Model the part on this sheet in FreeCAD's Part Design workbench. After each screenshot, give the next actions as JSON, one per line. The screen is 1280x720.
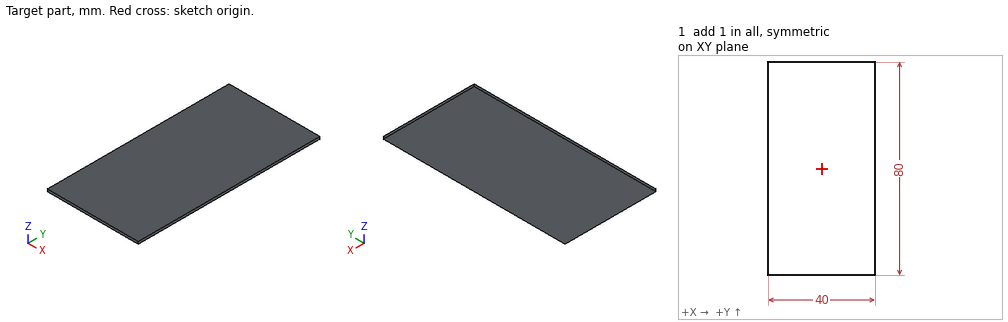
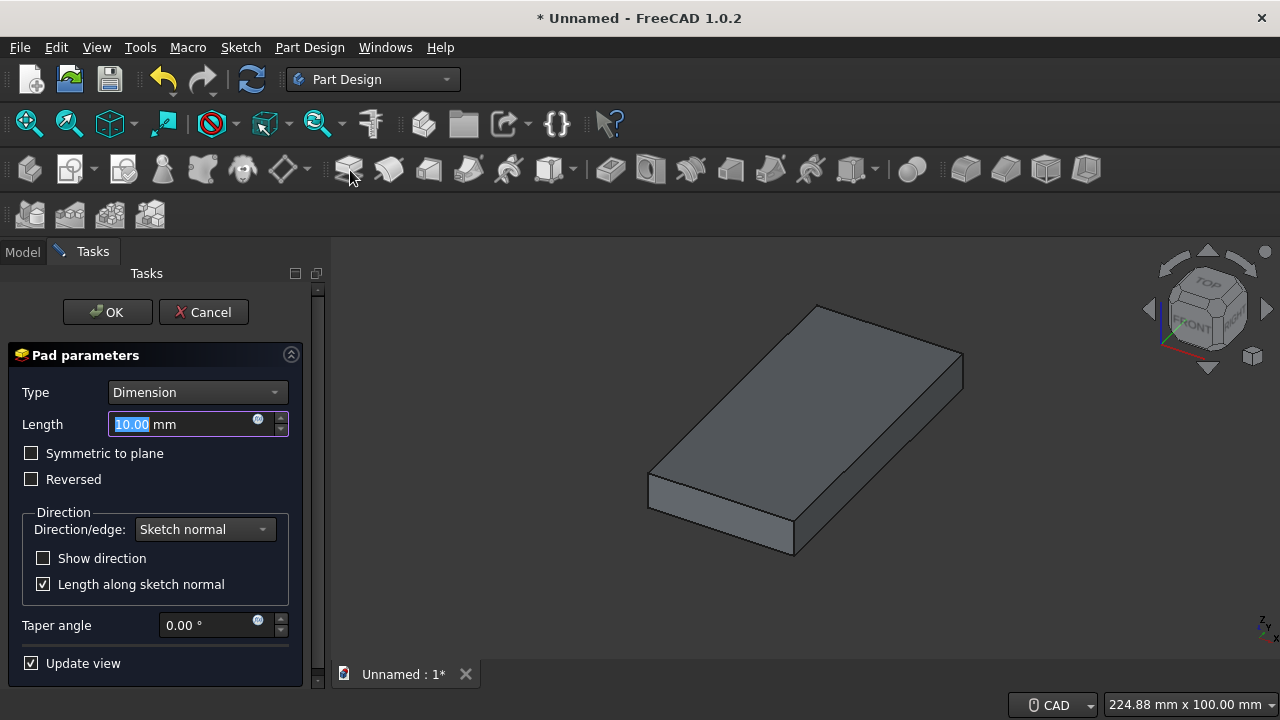
{"action": "type", "text": "1"}
{"action": "key", "text": "Tab"}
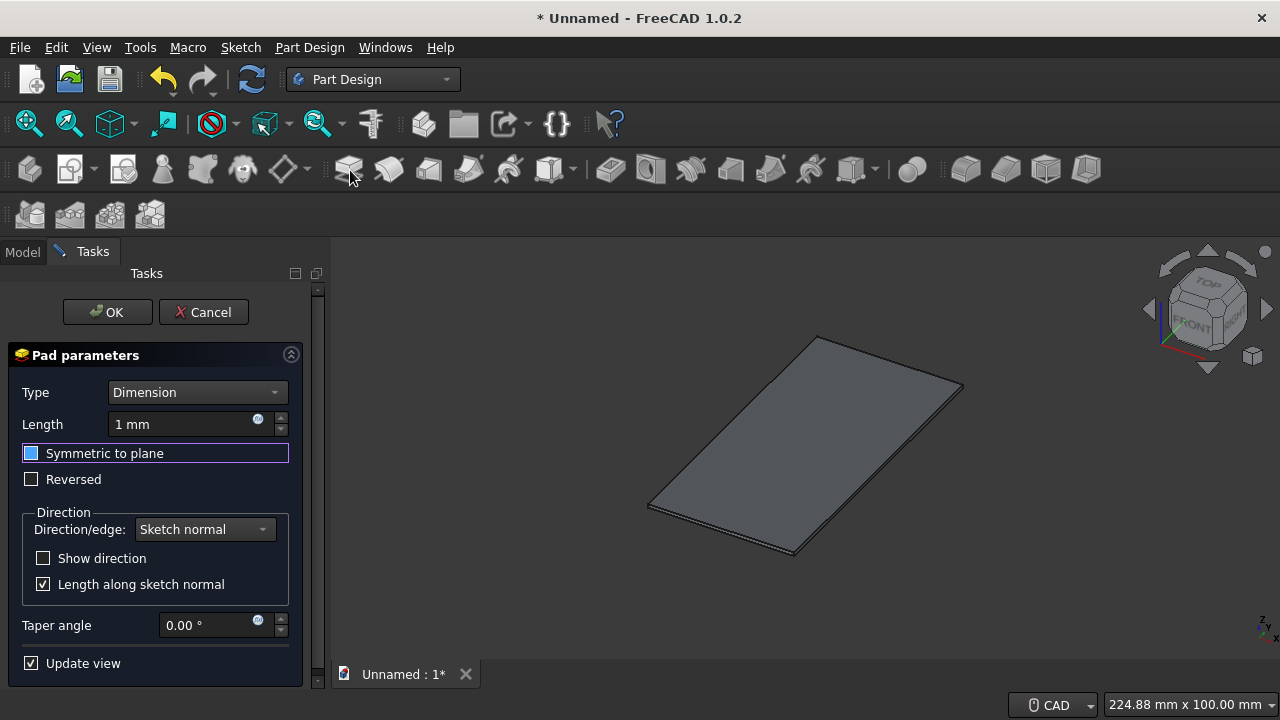
{"action": "left_click", "coordinate": [30, 453]}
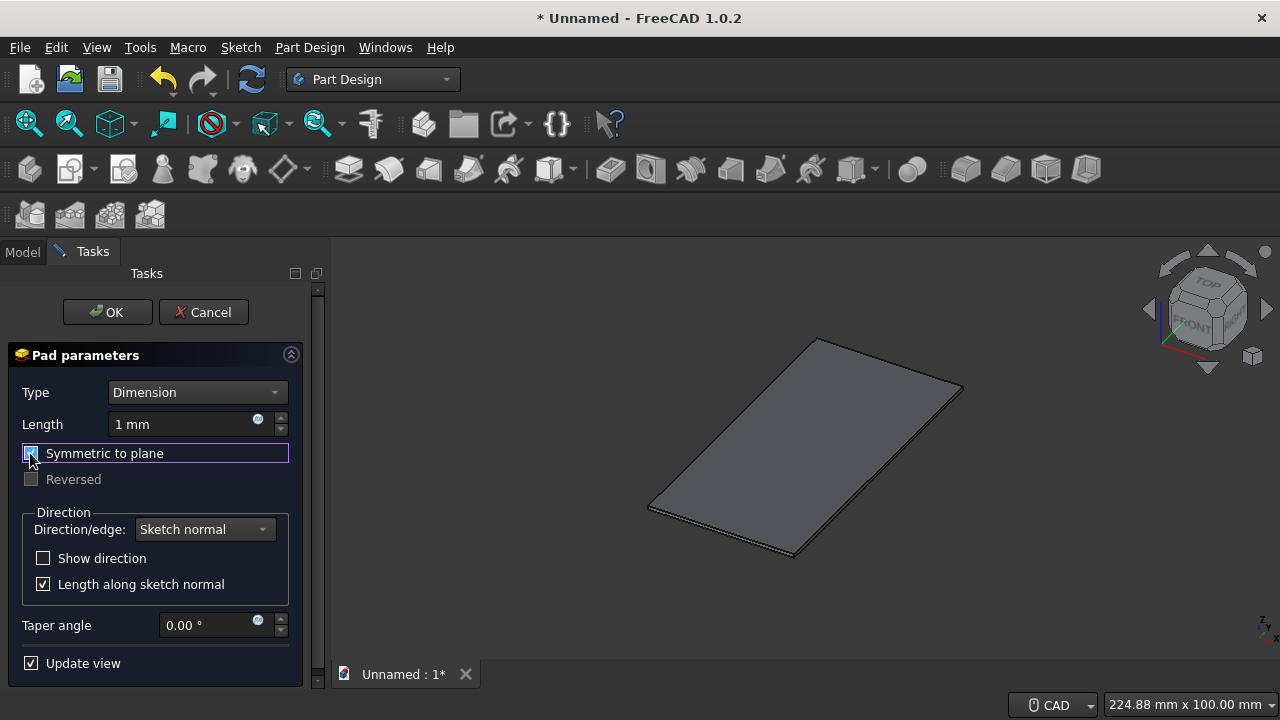
{"action": "left_click", "coordinate": [108, 312]}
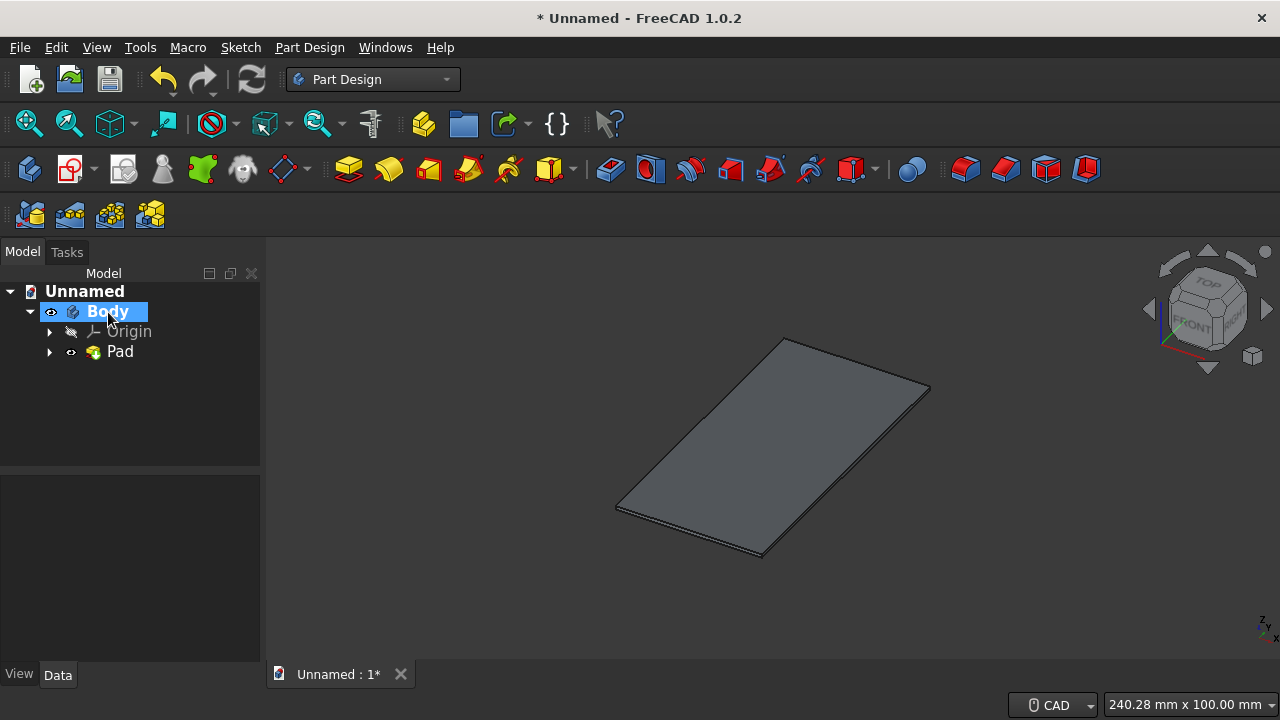
{"action": "key", "text": "0"}